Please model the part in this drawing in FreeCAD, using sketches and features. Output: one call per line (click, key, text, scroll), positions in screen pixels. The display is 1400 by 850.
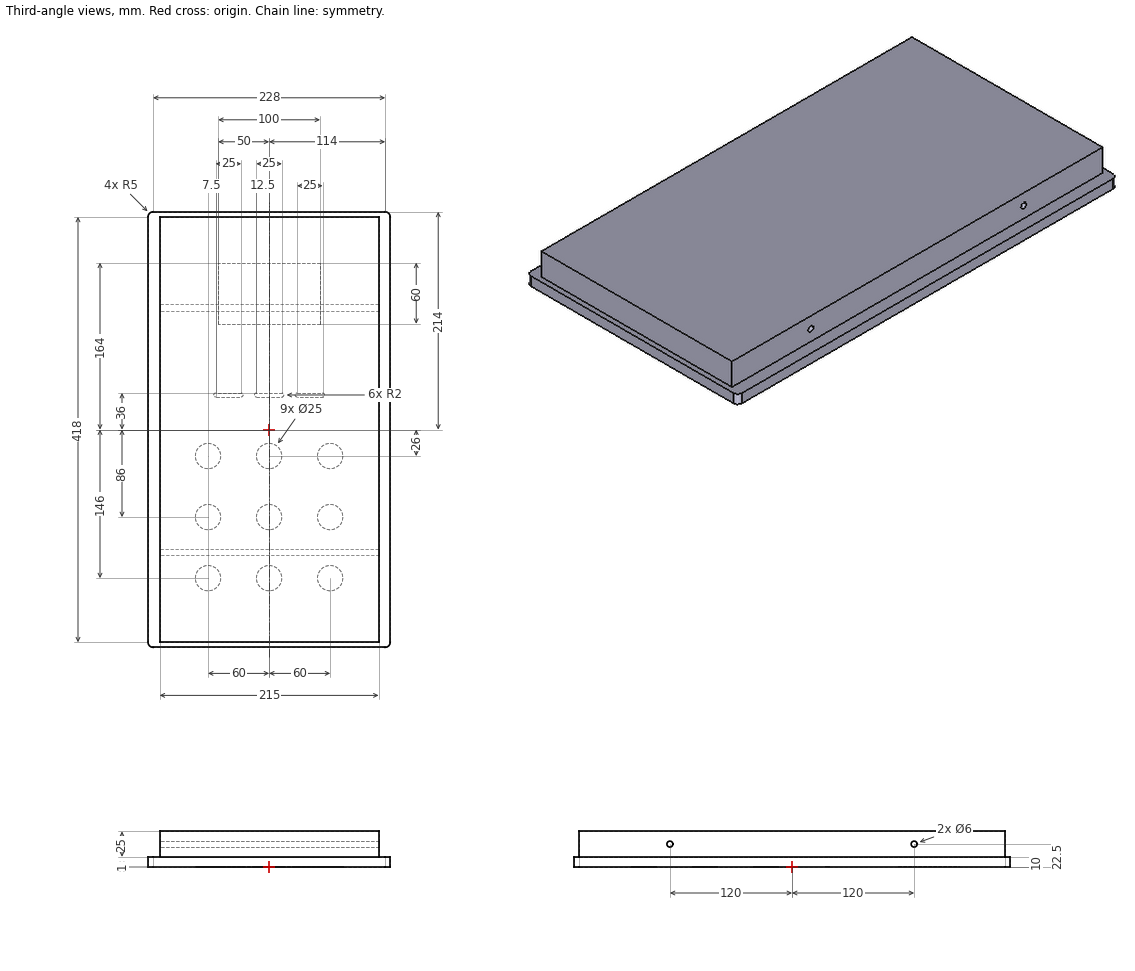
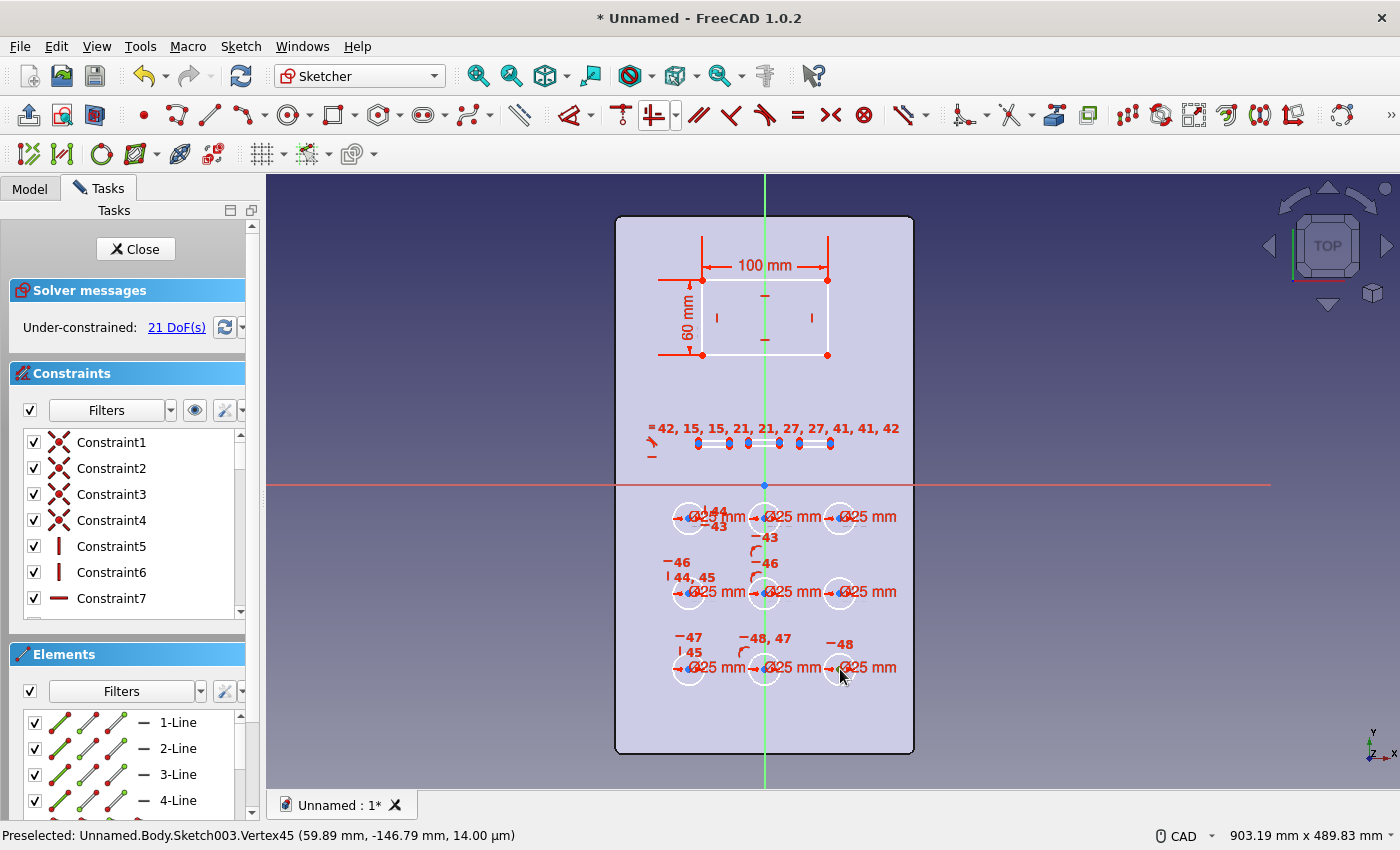
click(840, 594)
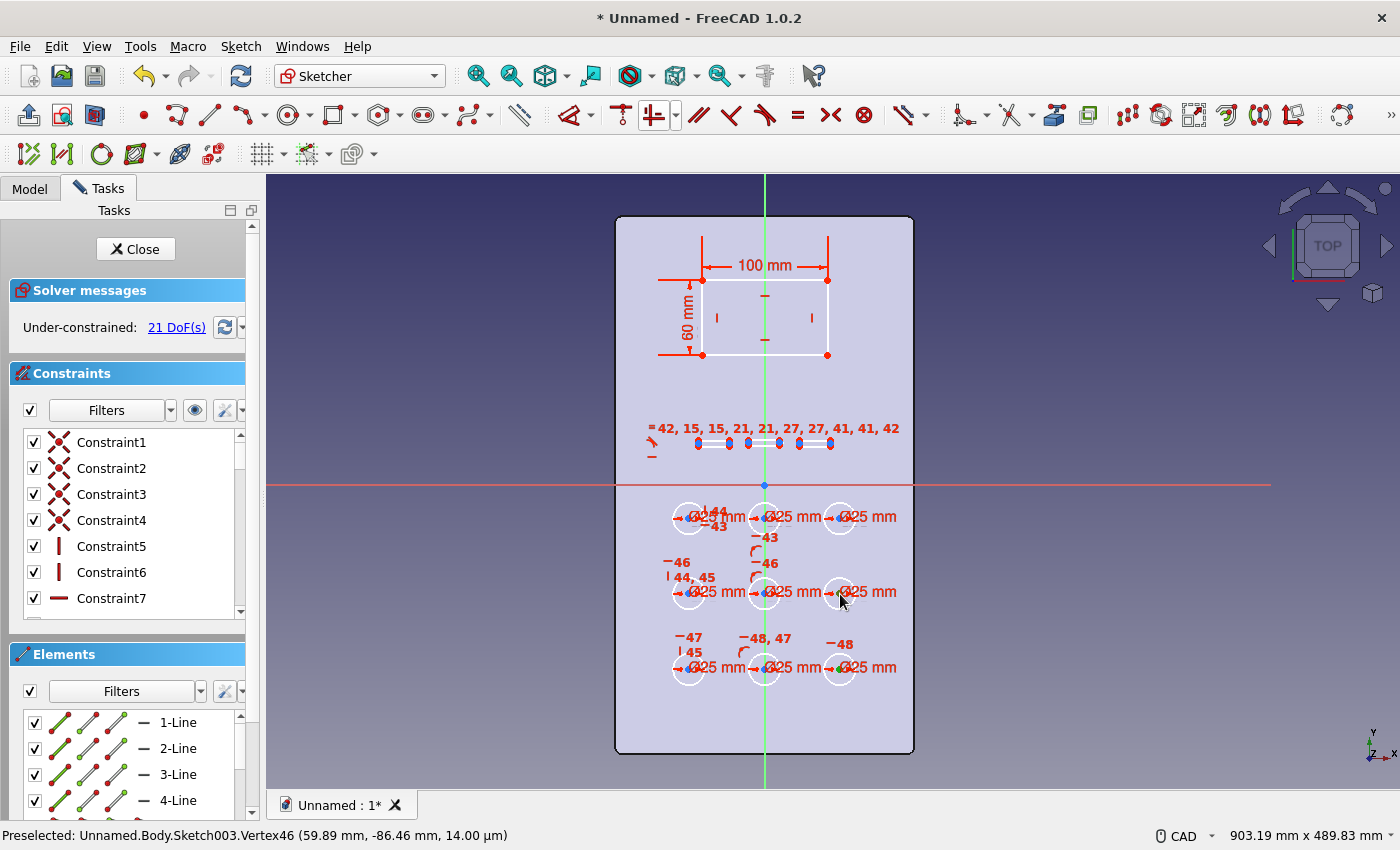
key(v)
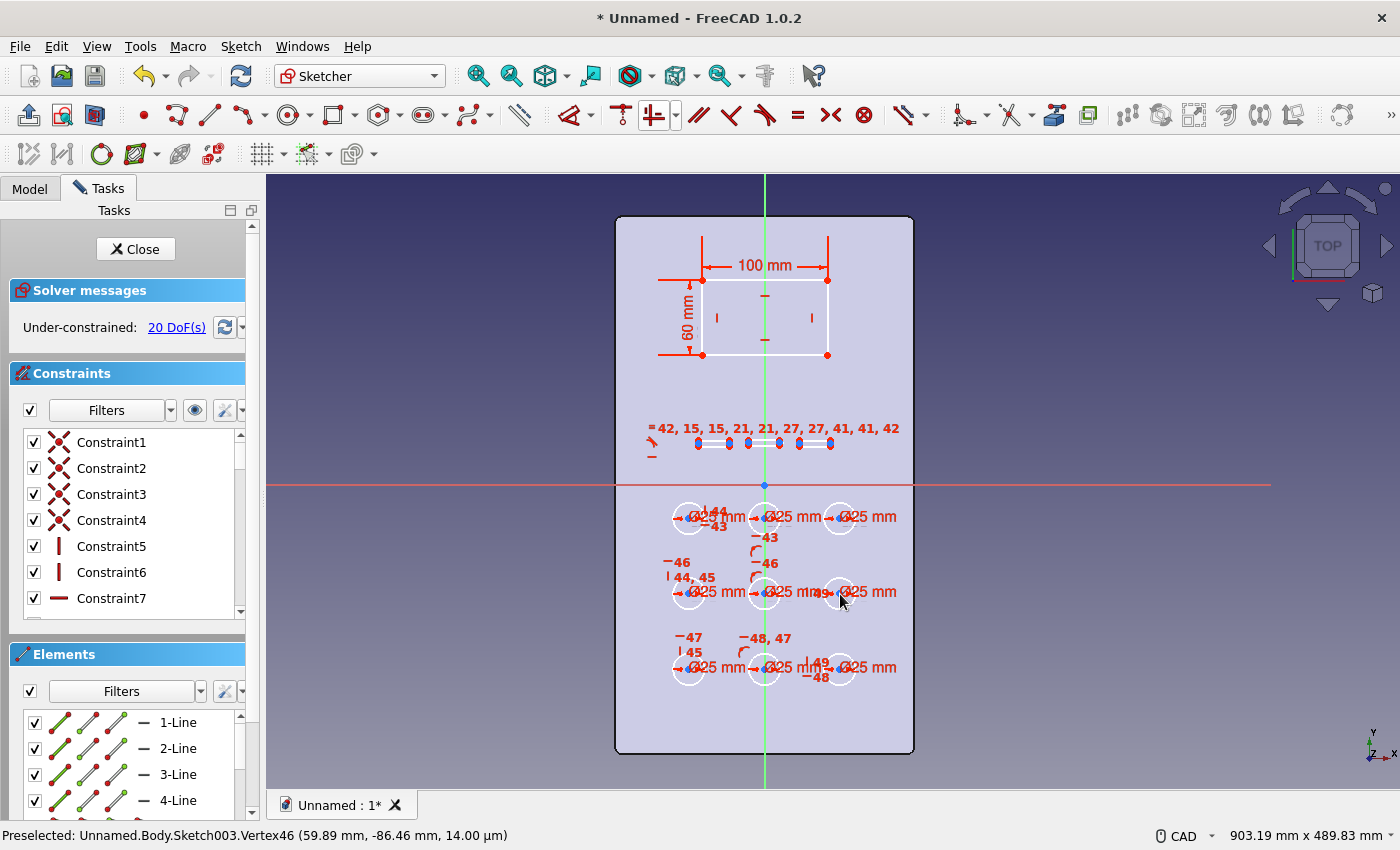
click(765, 594)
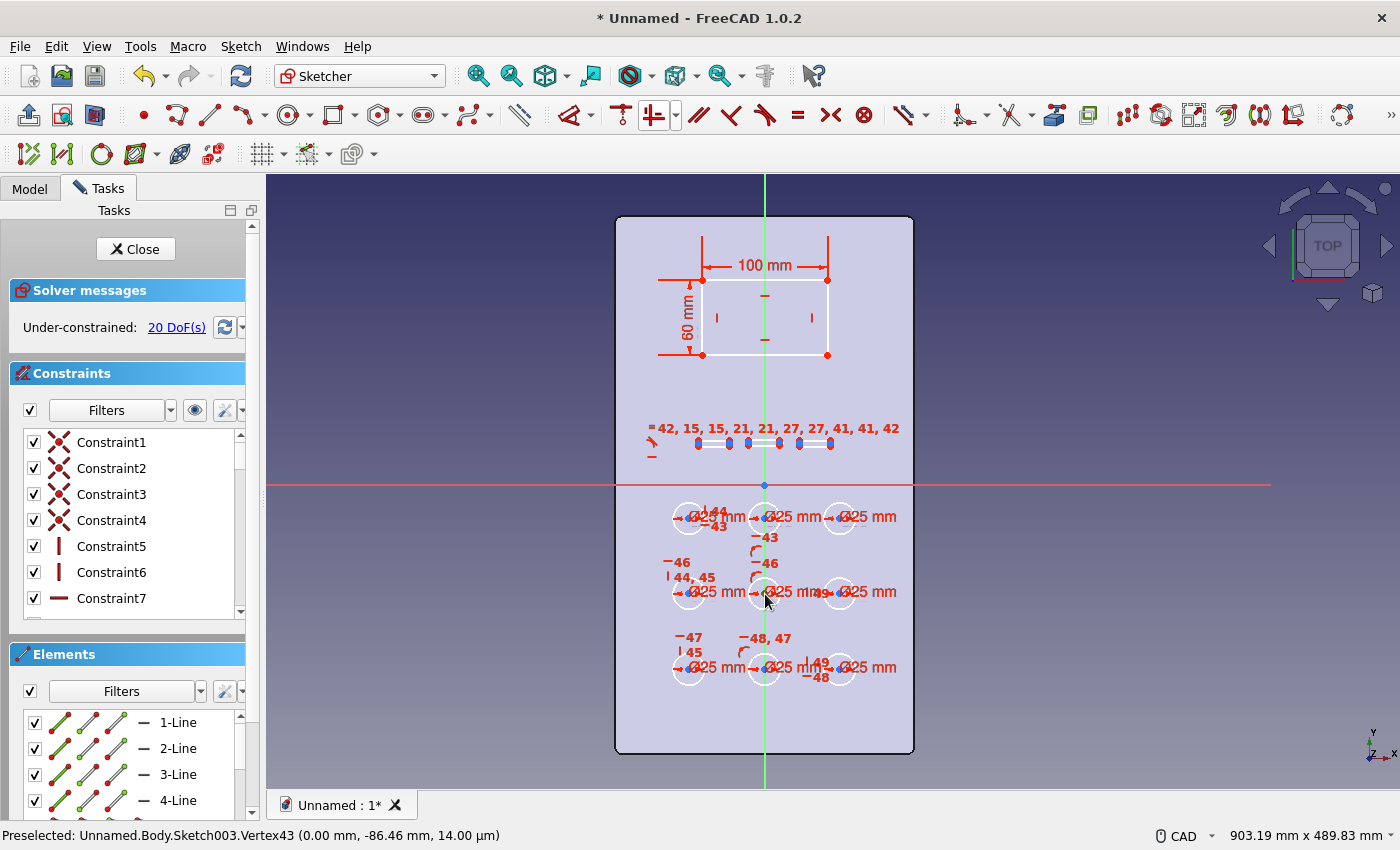
click(840, 594)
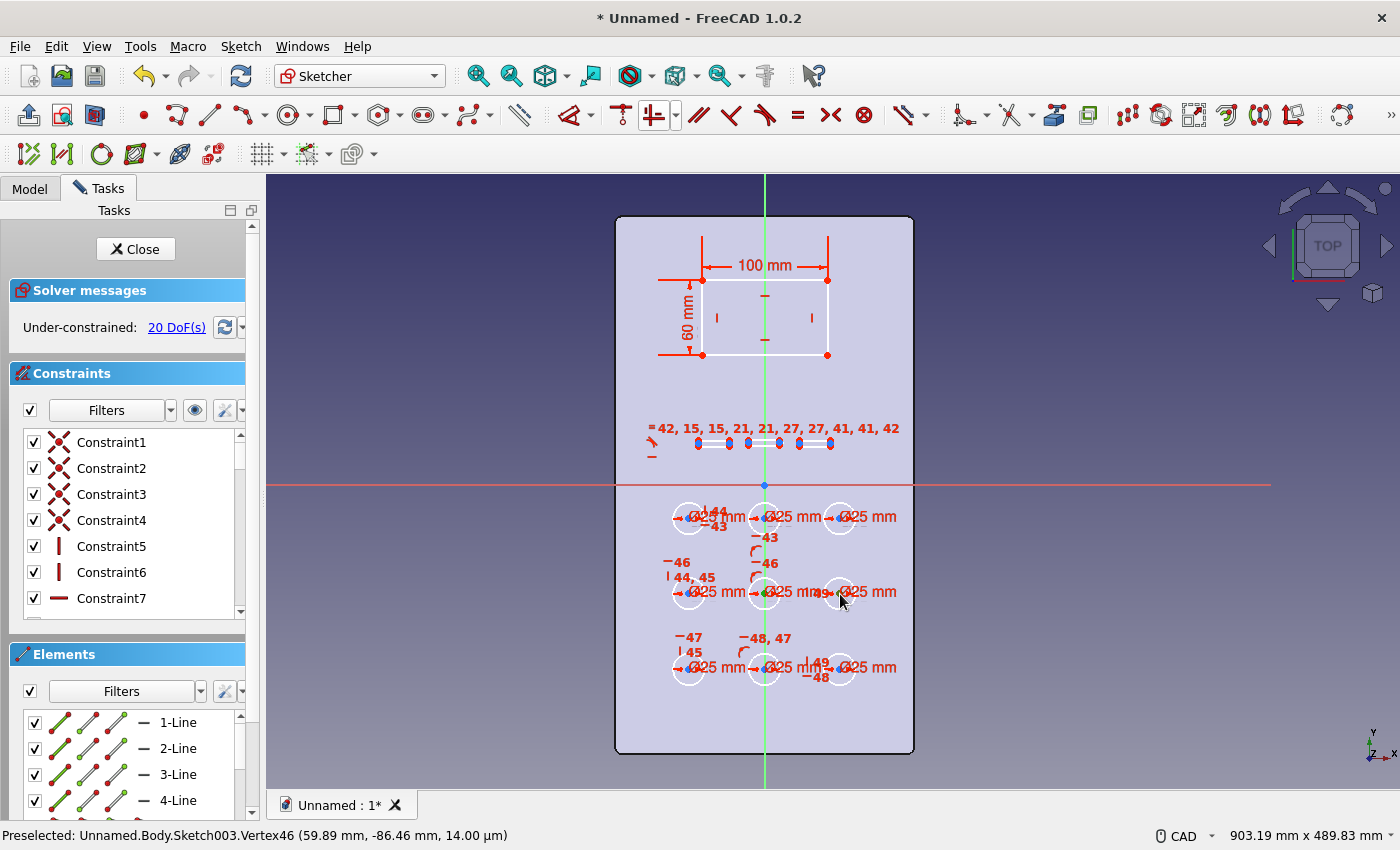
click(676, 116)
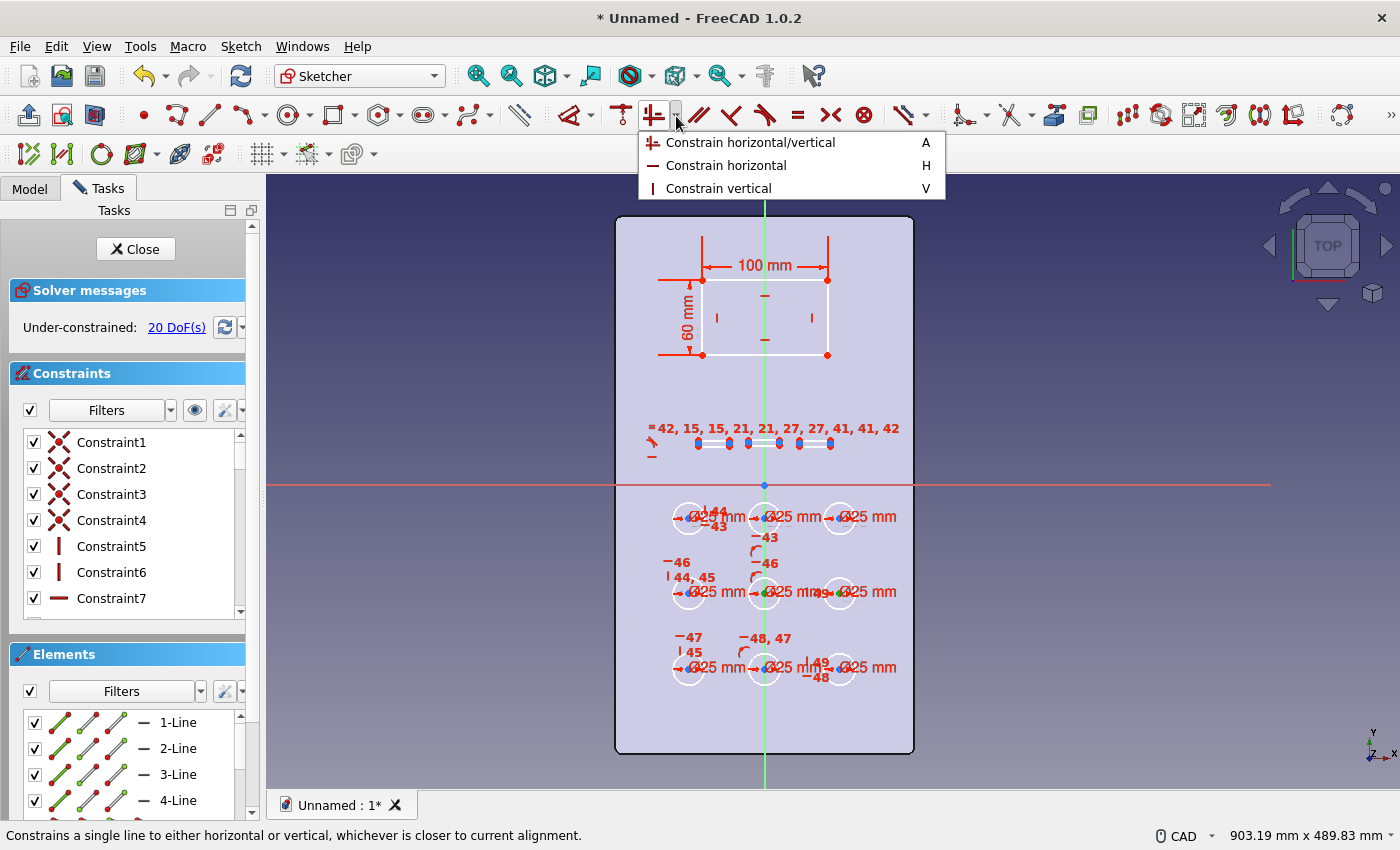
click(792, 166)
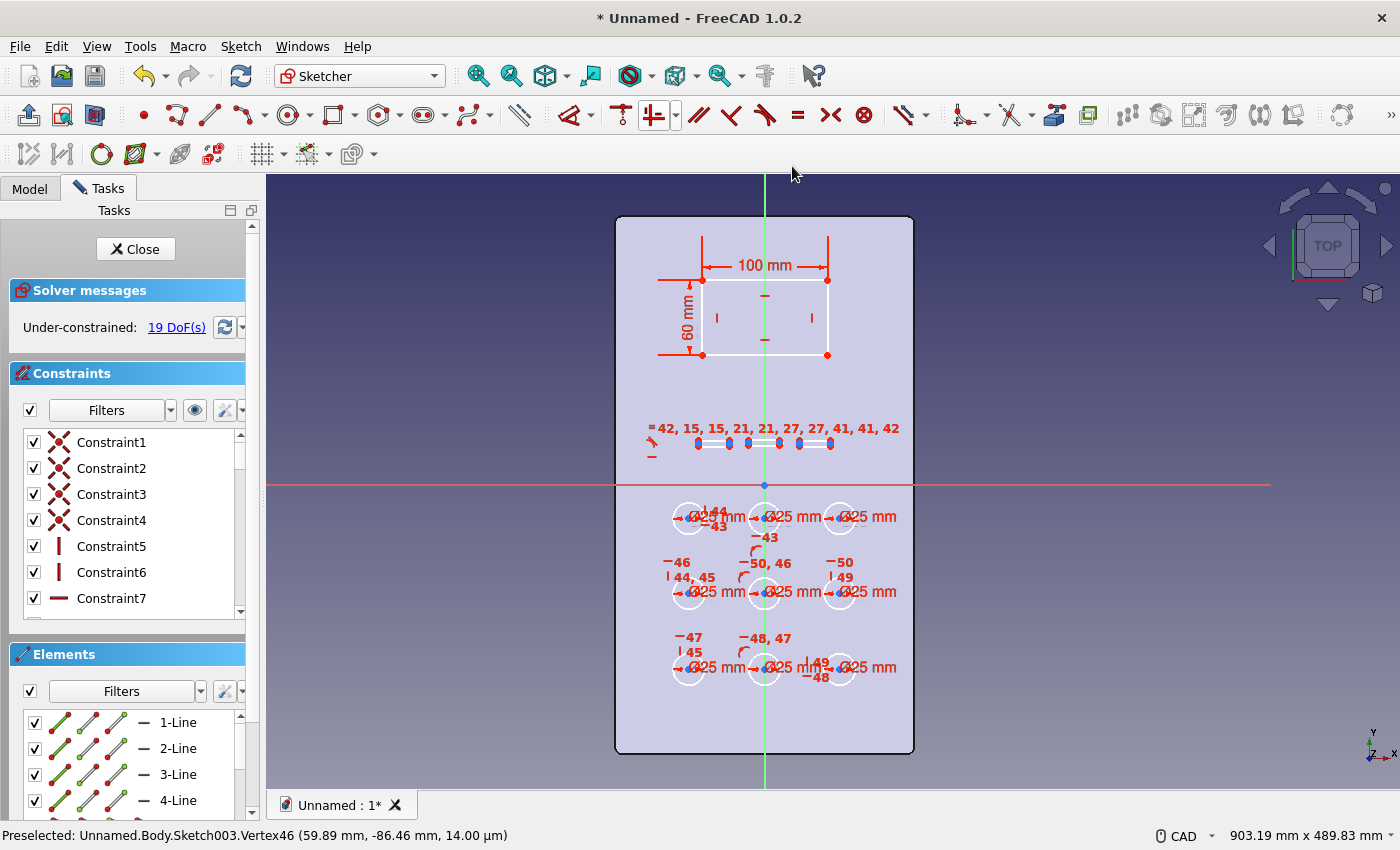
click(840, 594)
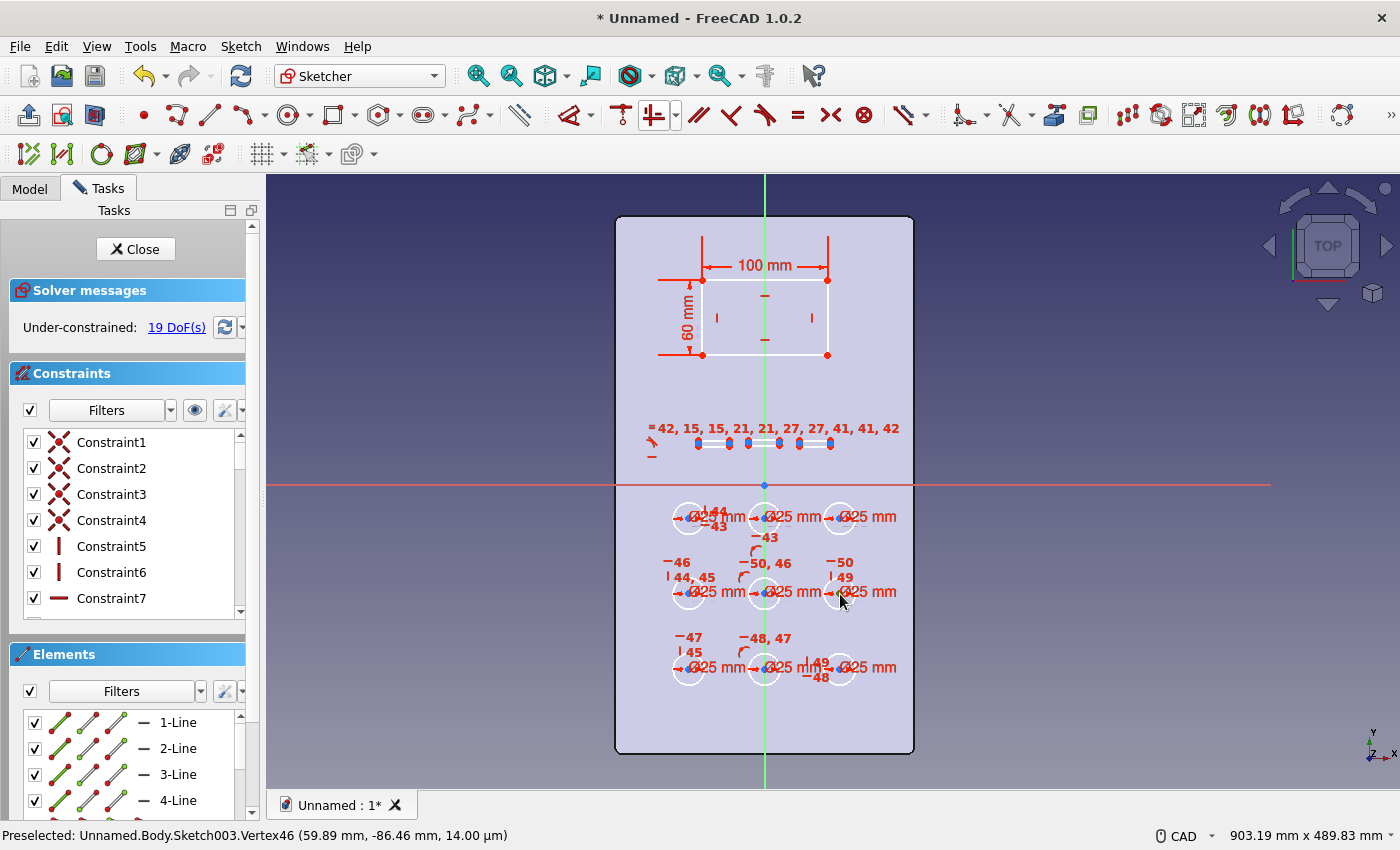
click(840, 519)